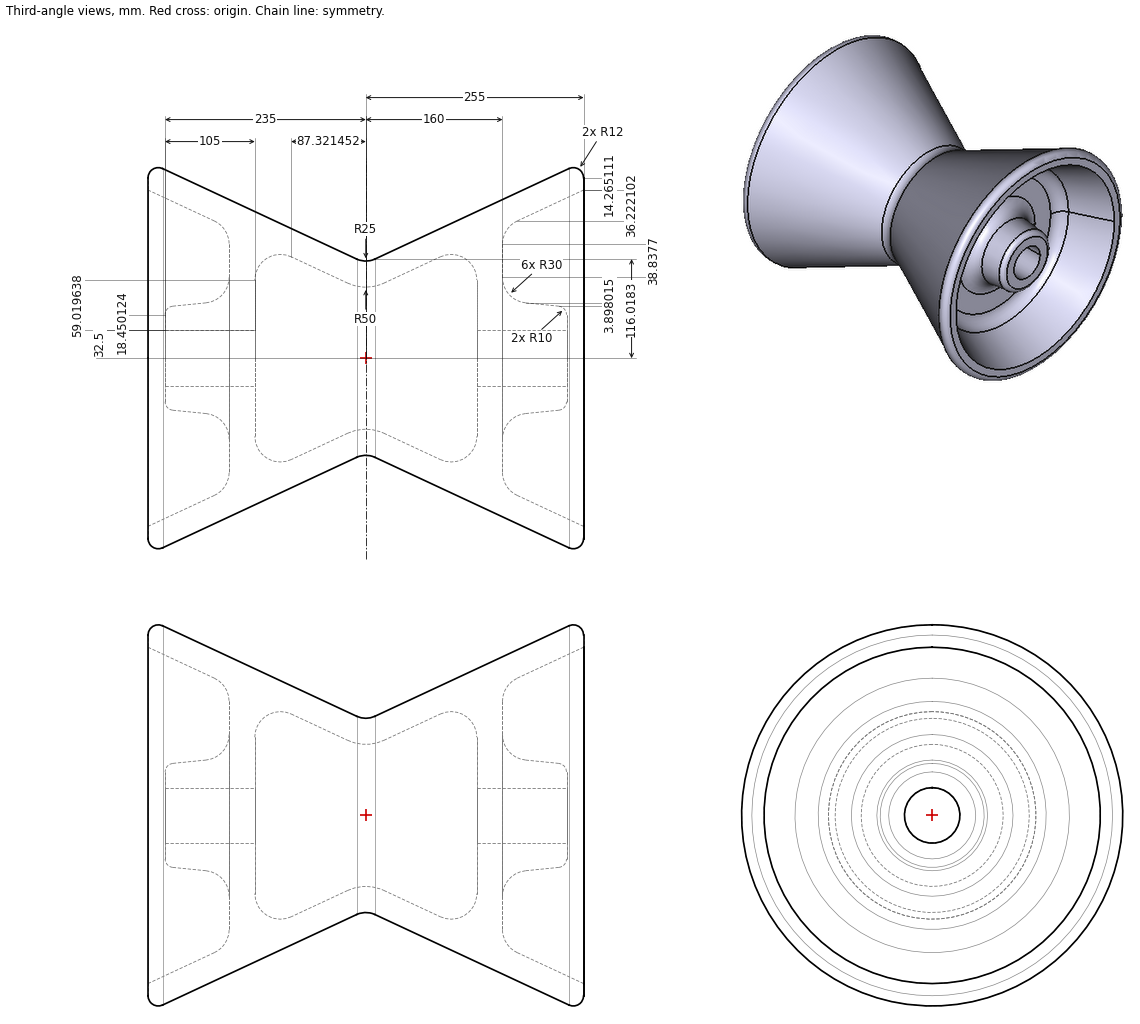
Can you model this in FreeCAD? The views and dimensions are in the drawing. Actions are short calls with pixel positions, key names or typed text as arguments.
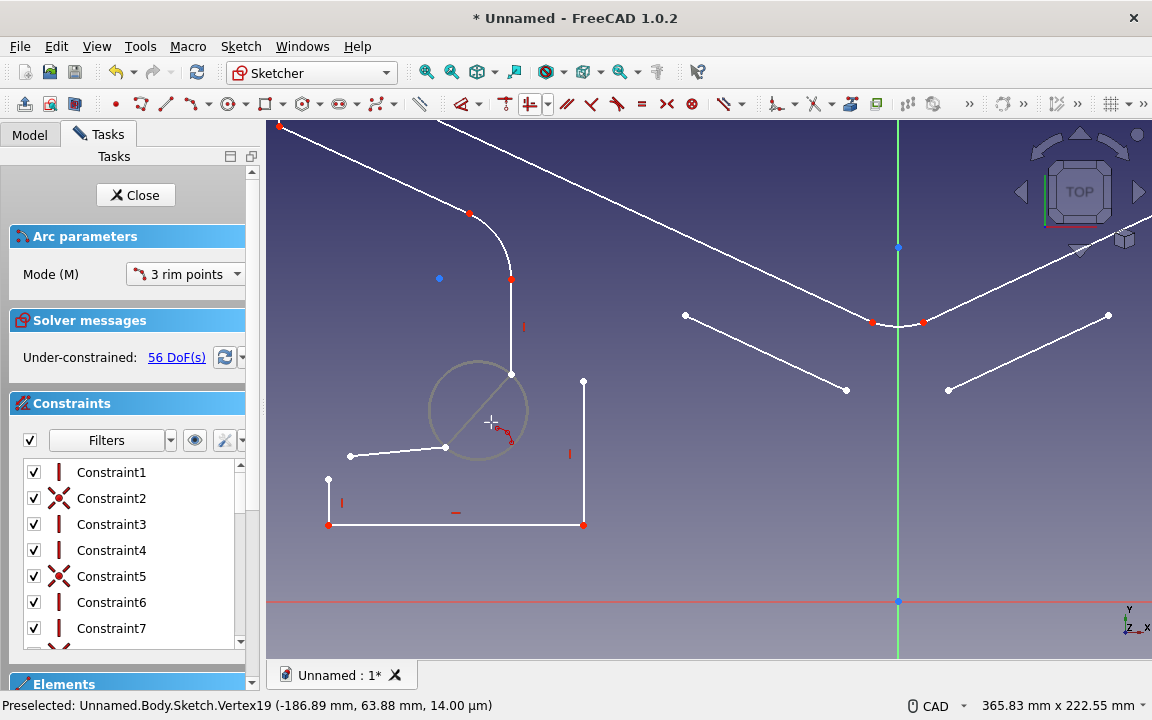
click(492, 421)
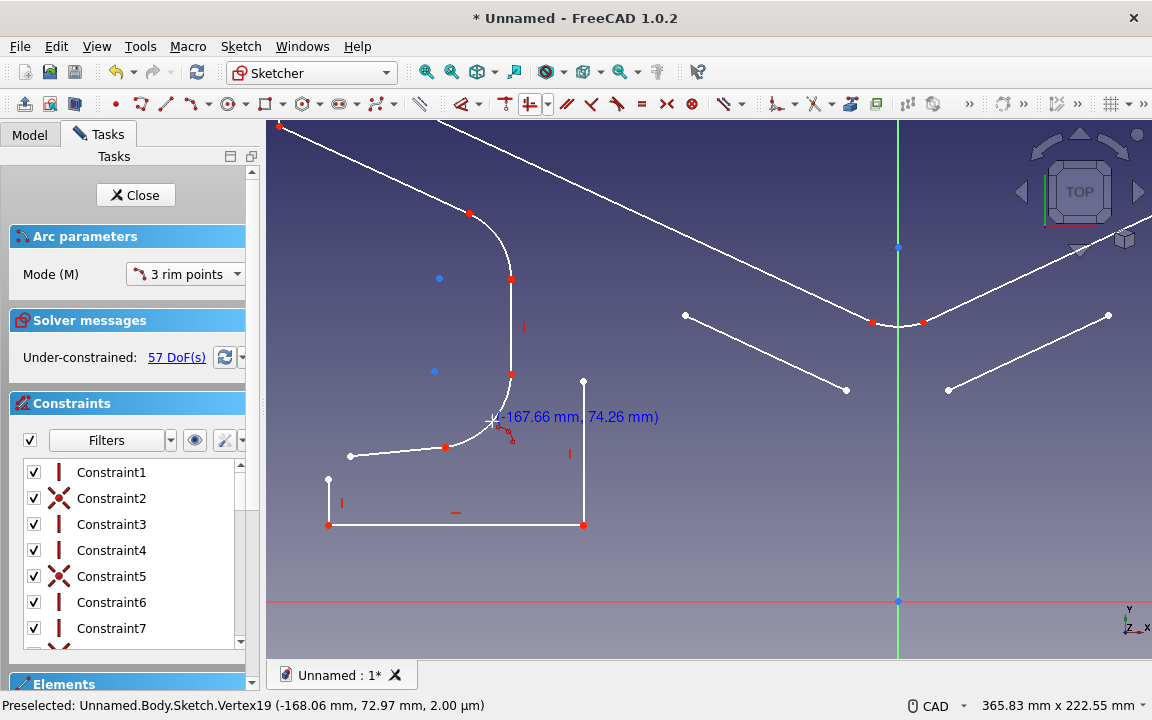
click(351, 456)
click(329, 480)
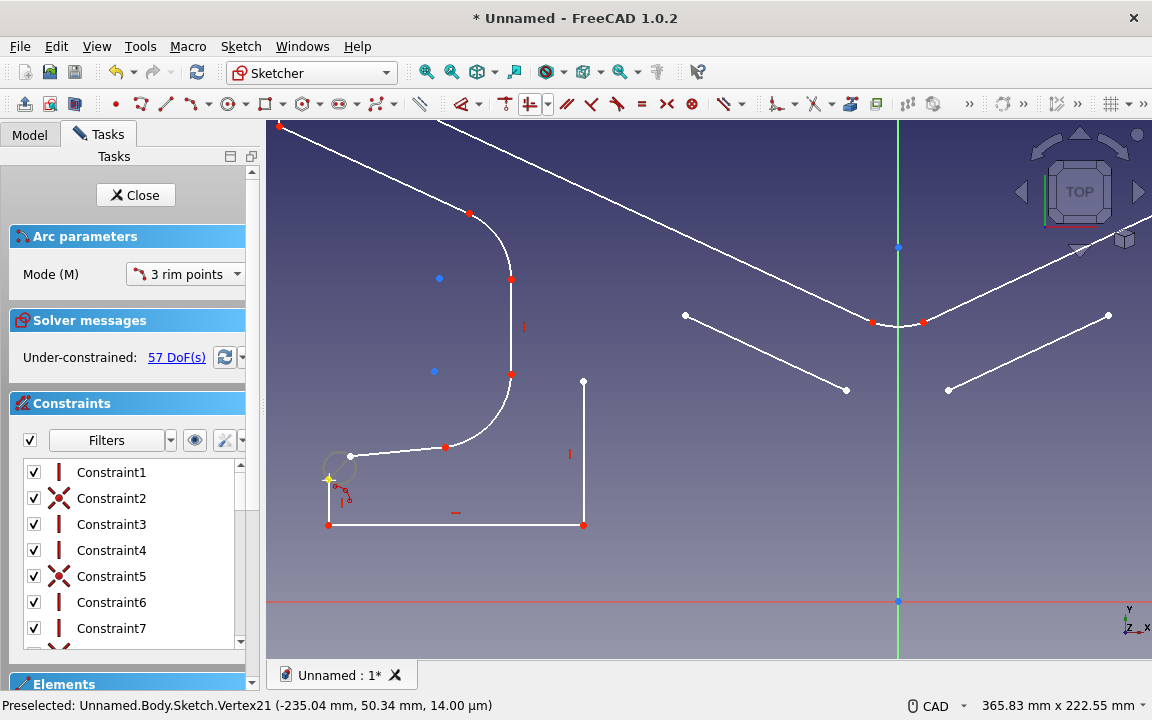
scroll(335, 462, up, 5)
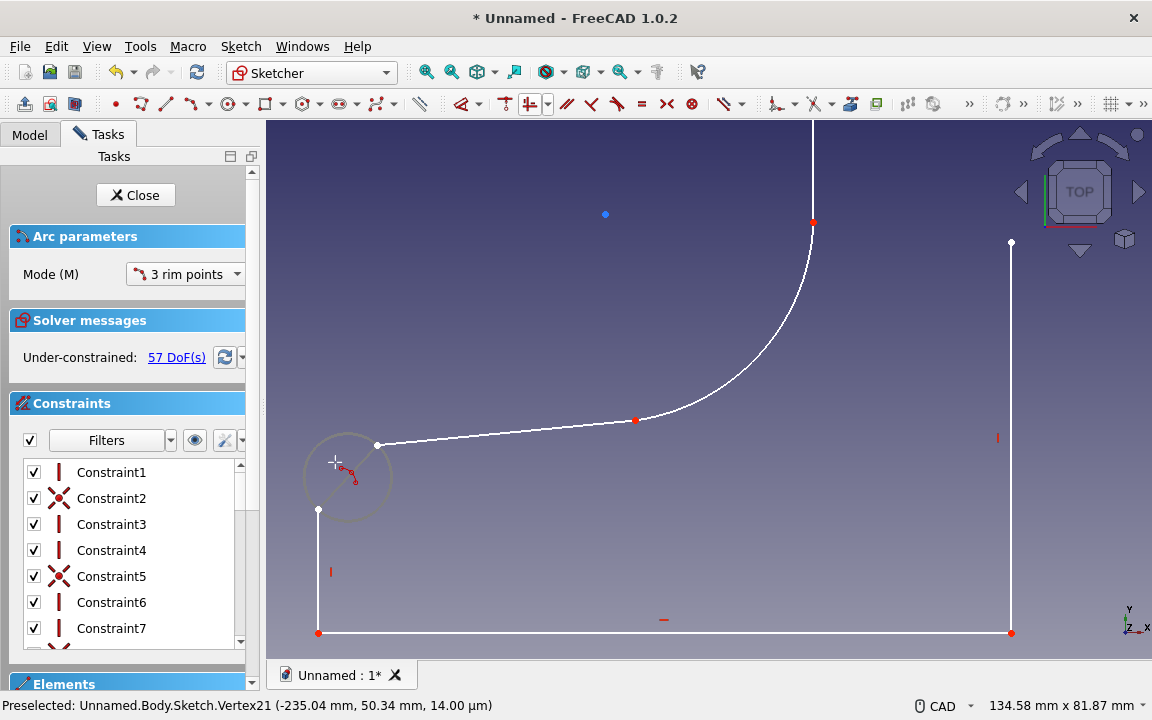
click(335, 461)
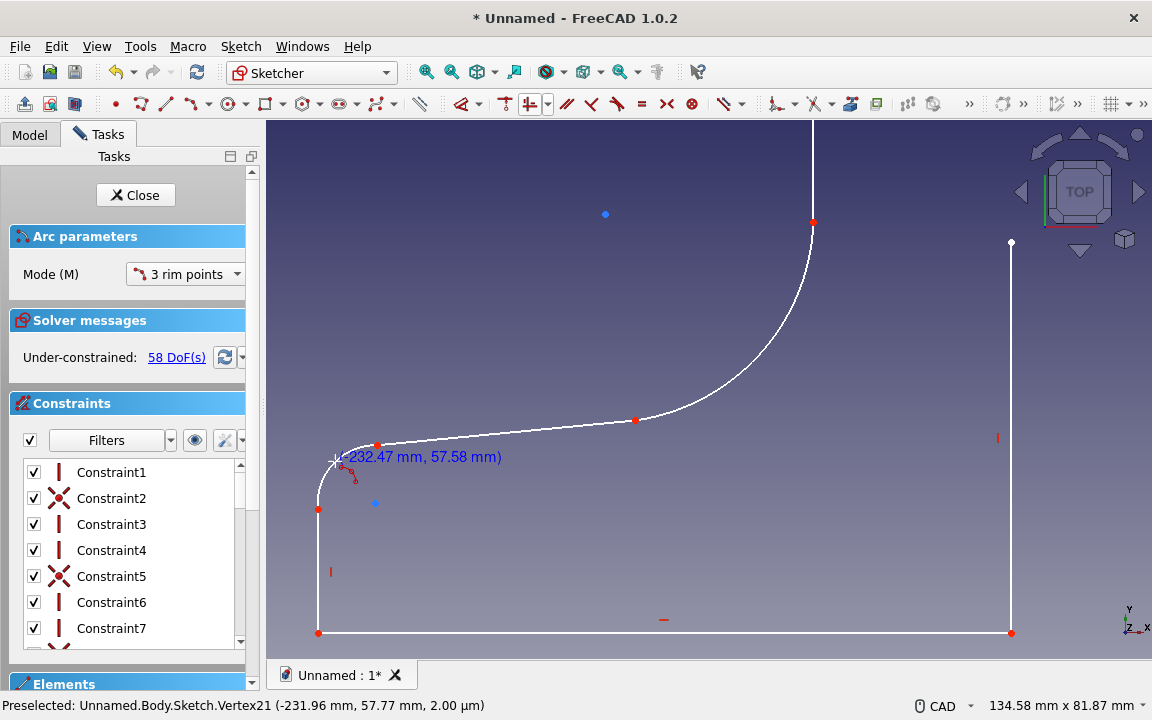
scroll(449, 433, down, 10)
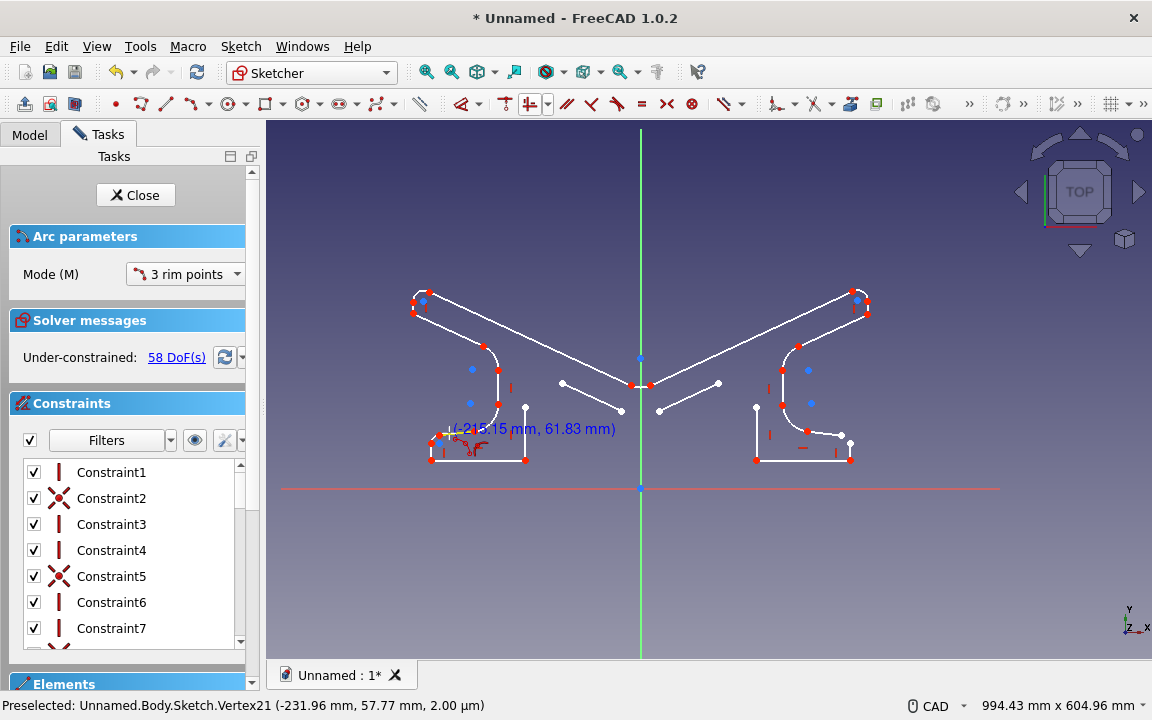
click(525, 408)
click(563, 384)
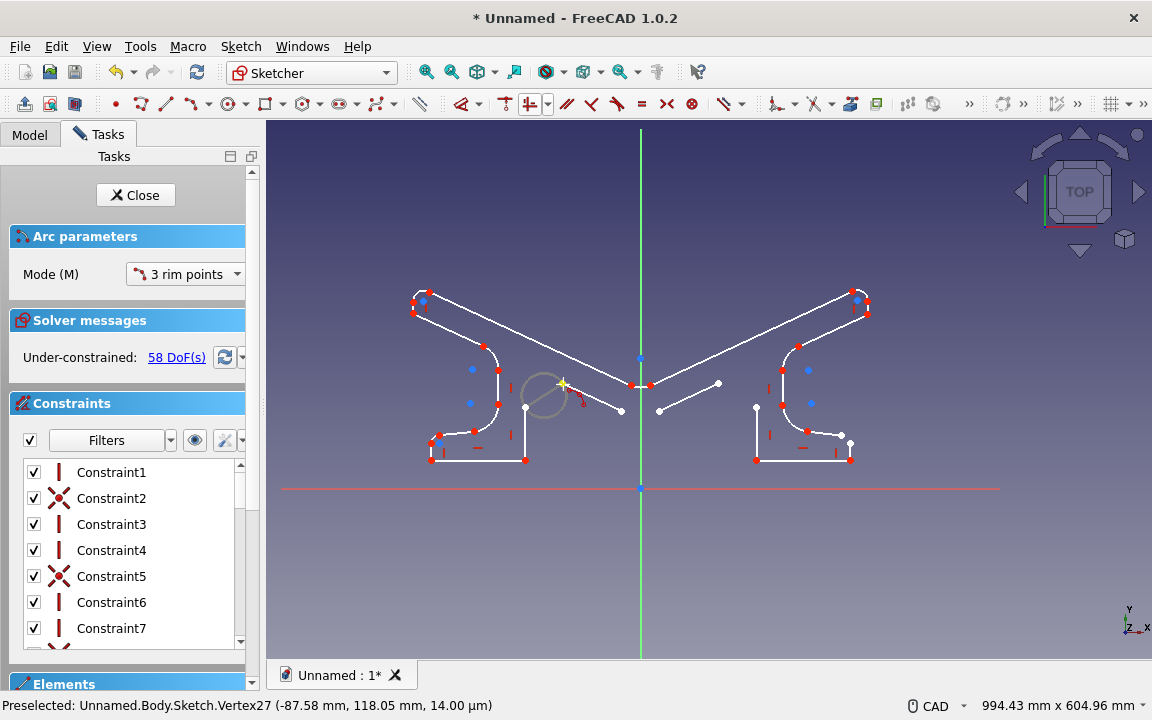
scroll(537, 385, up, 2)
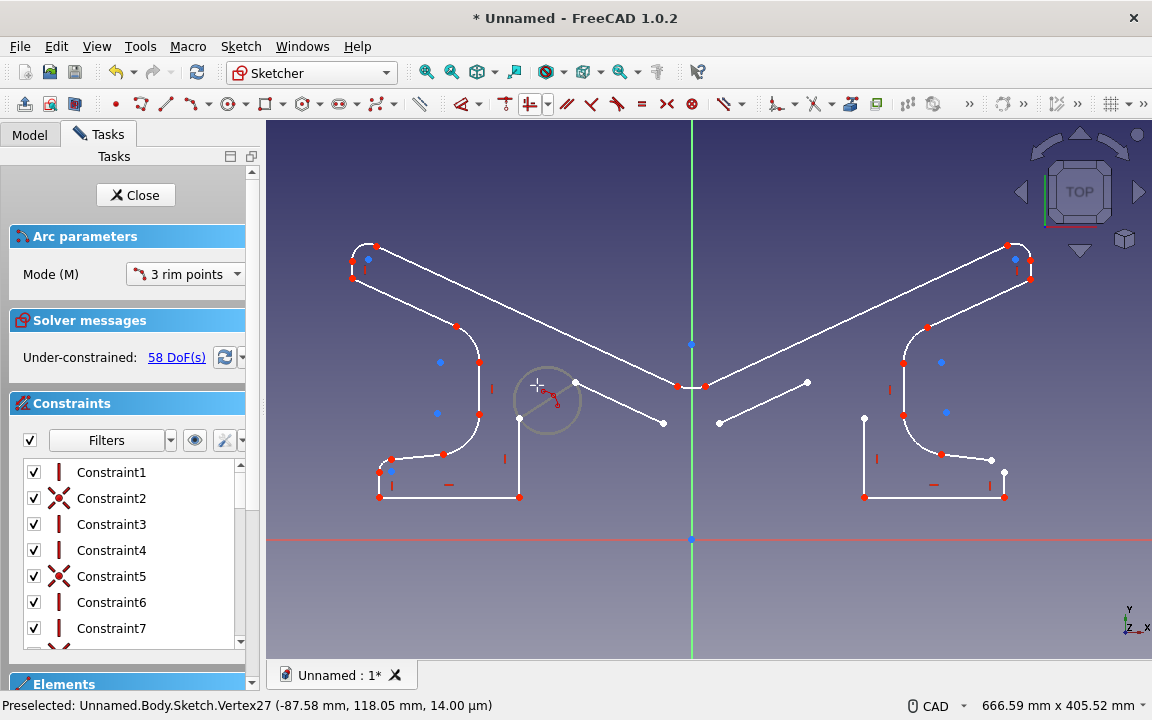
click(537, 384)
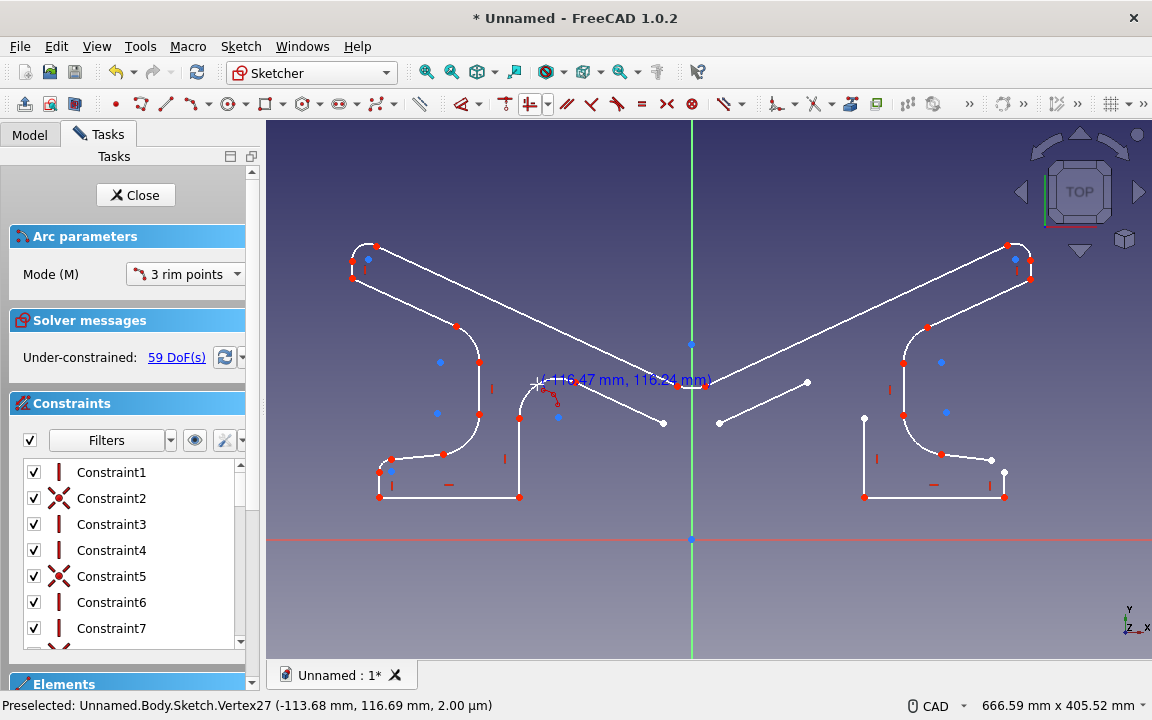
click(663, 424)
click(719, 424)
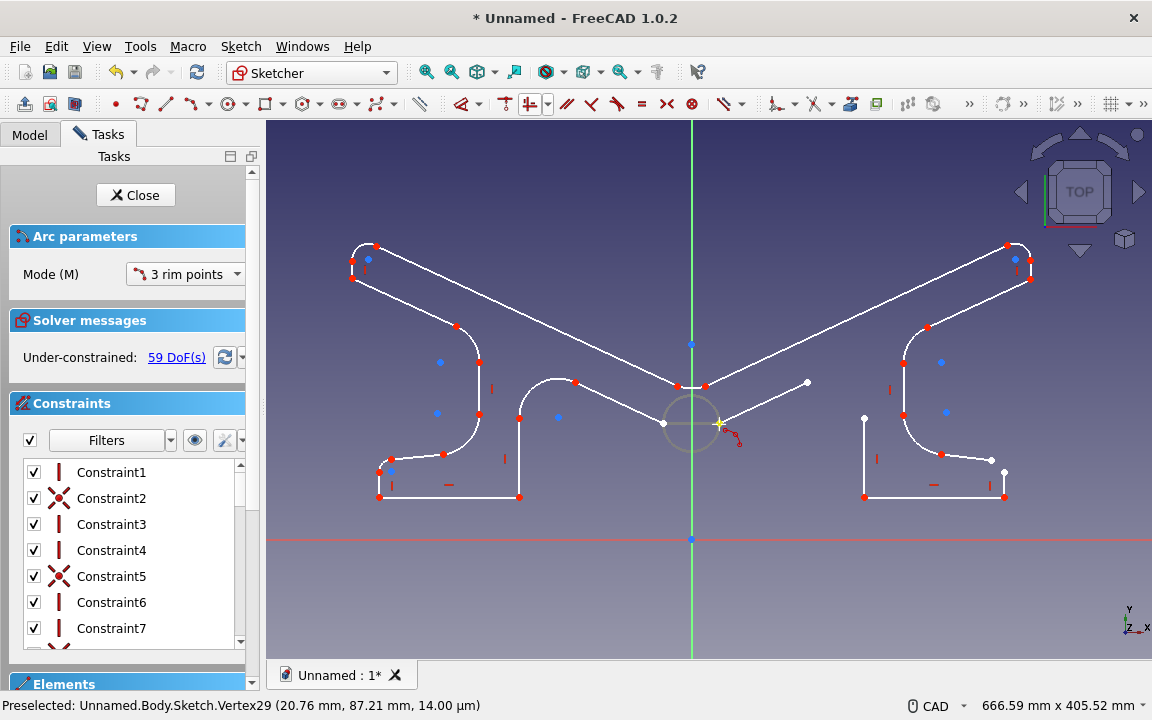
scroll(686, 429, up, 6)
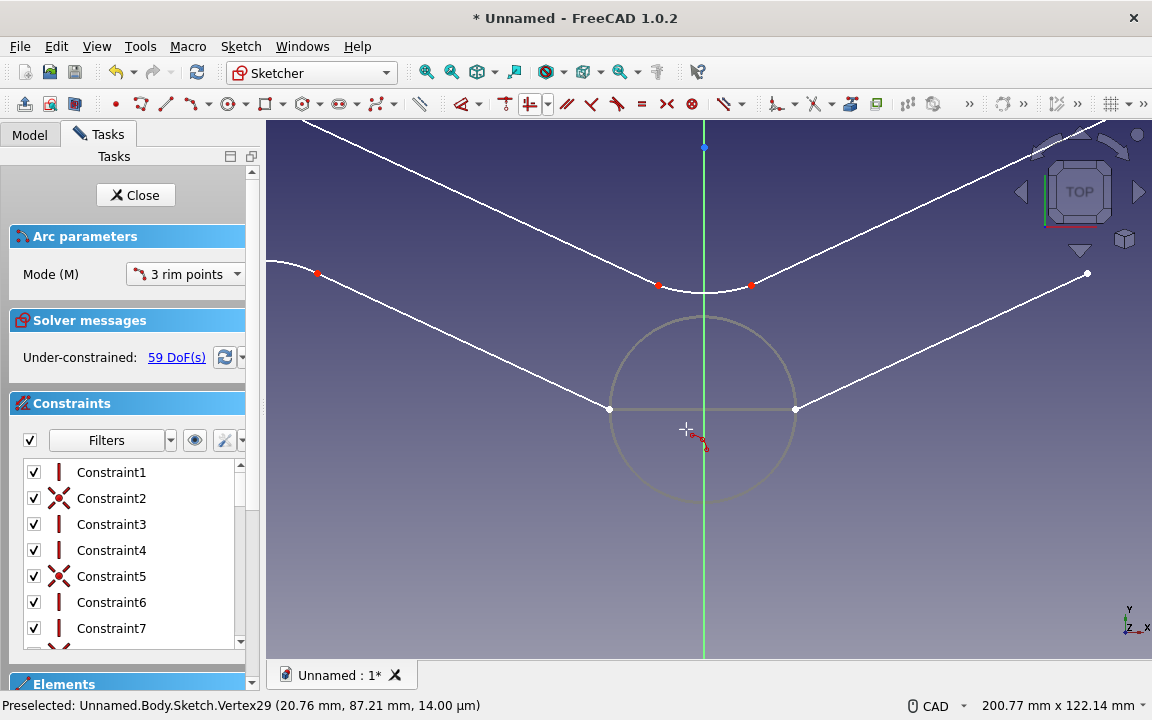
click(685, 427)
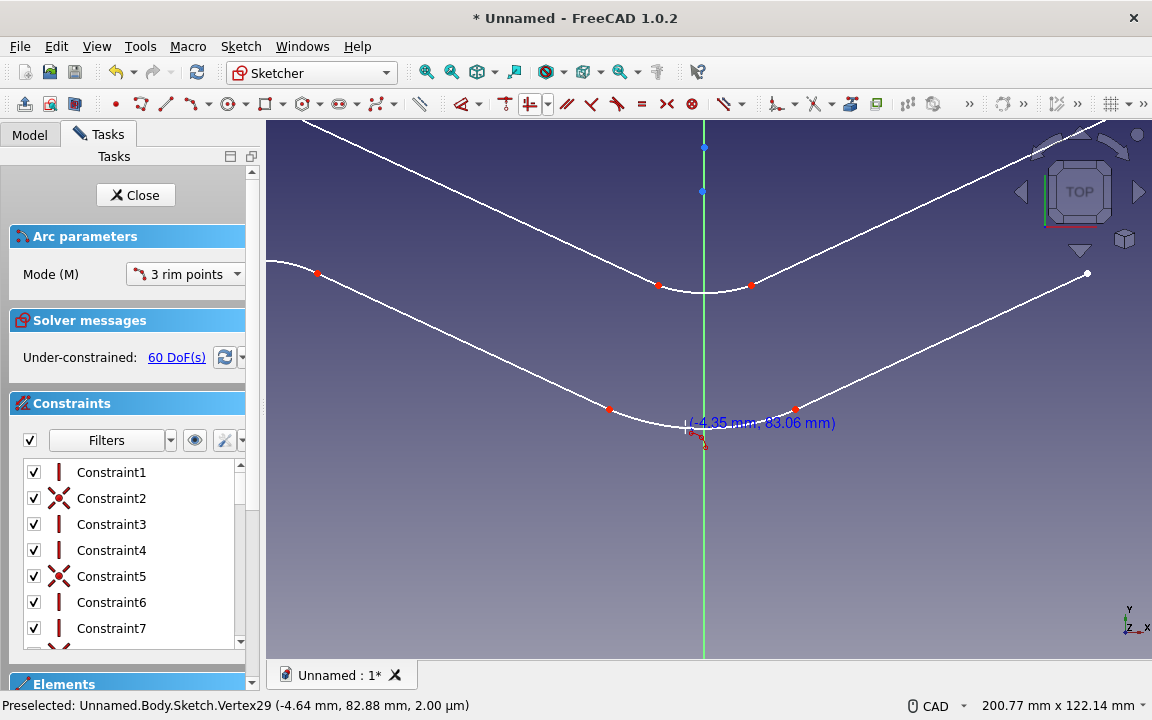
scroll(624, 411, down, 8)